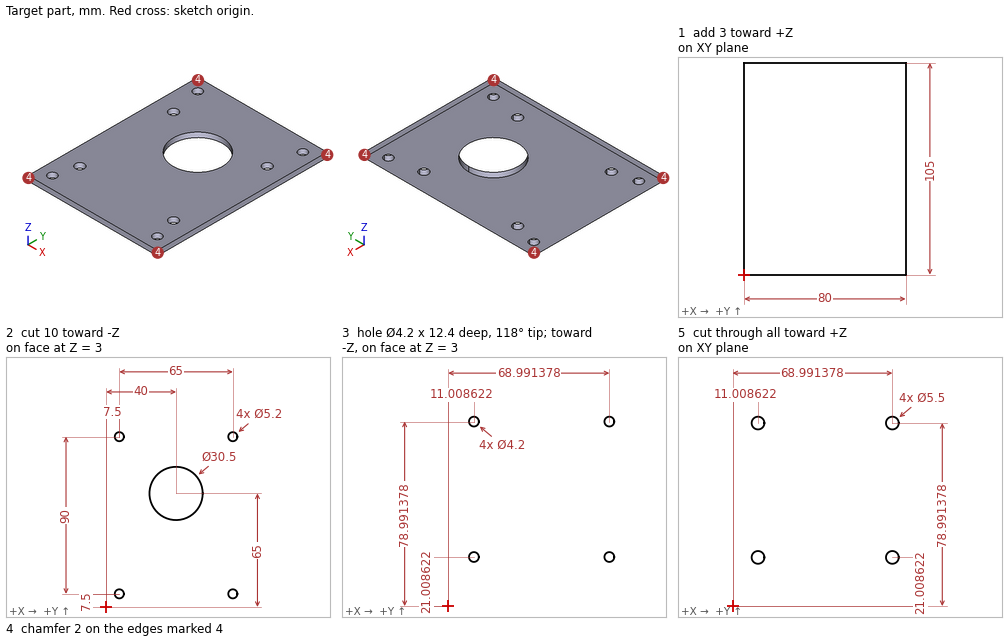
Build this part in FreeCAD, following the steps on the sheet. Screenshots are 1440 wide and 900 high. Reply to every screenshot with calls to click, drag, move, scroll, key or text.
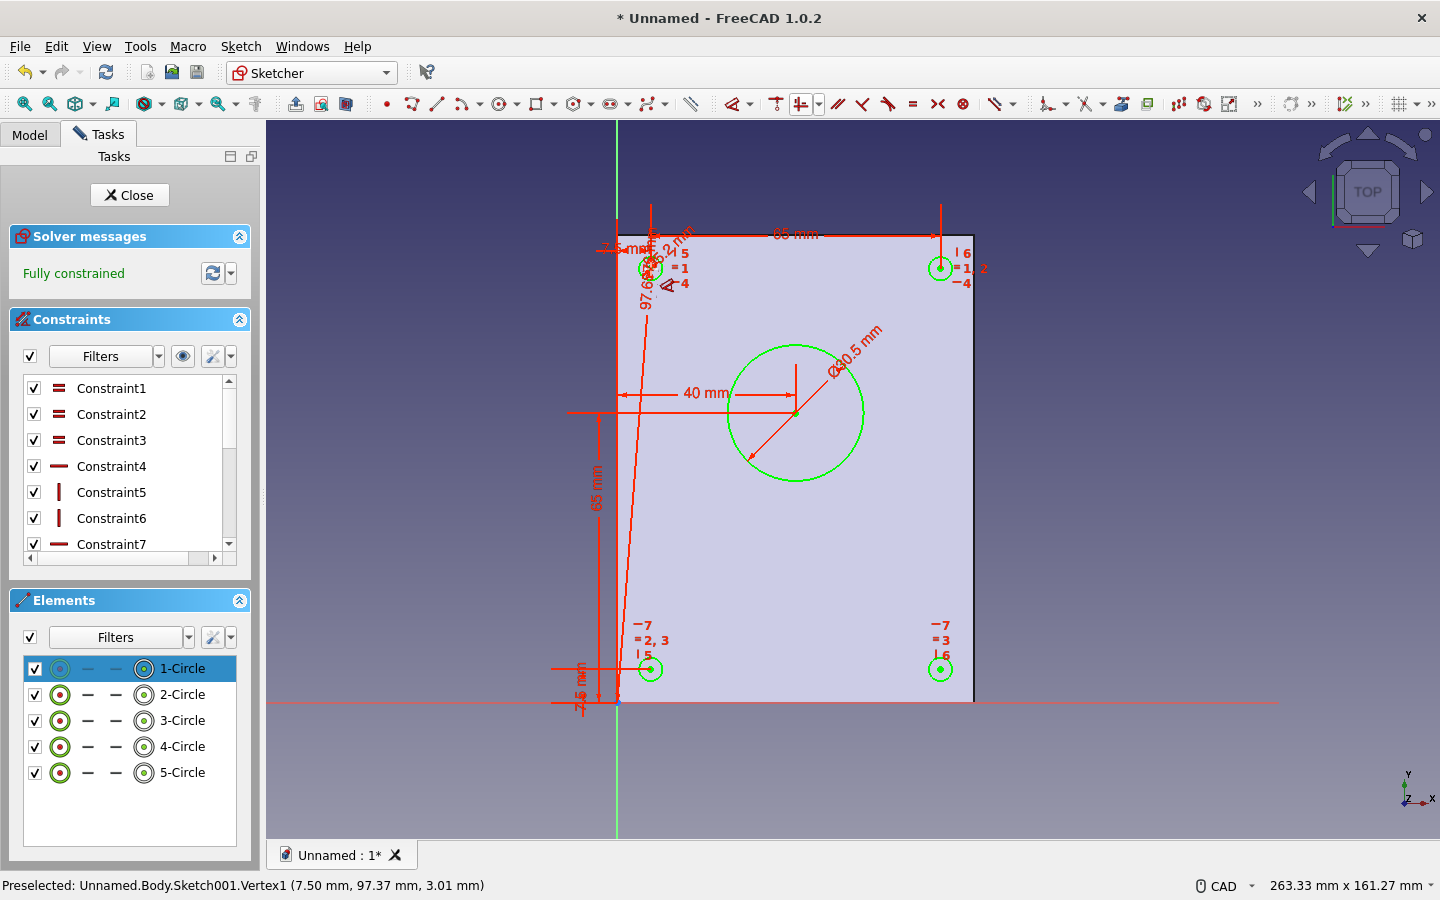
click(651, 669)
click(685, 469)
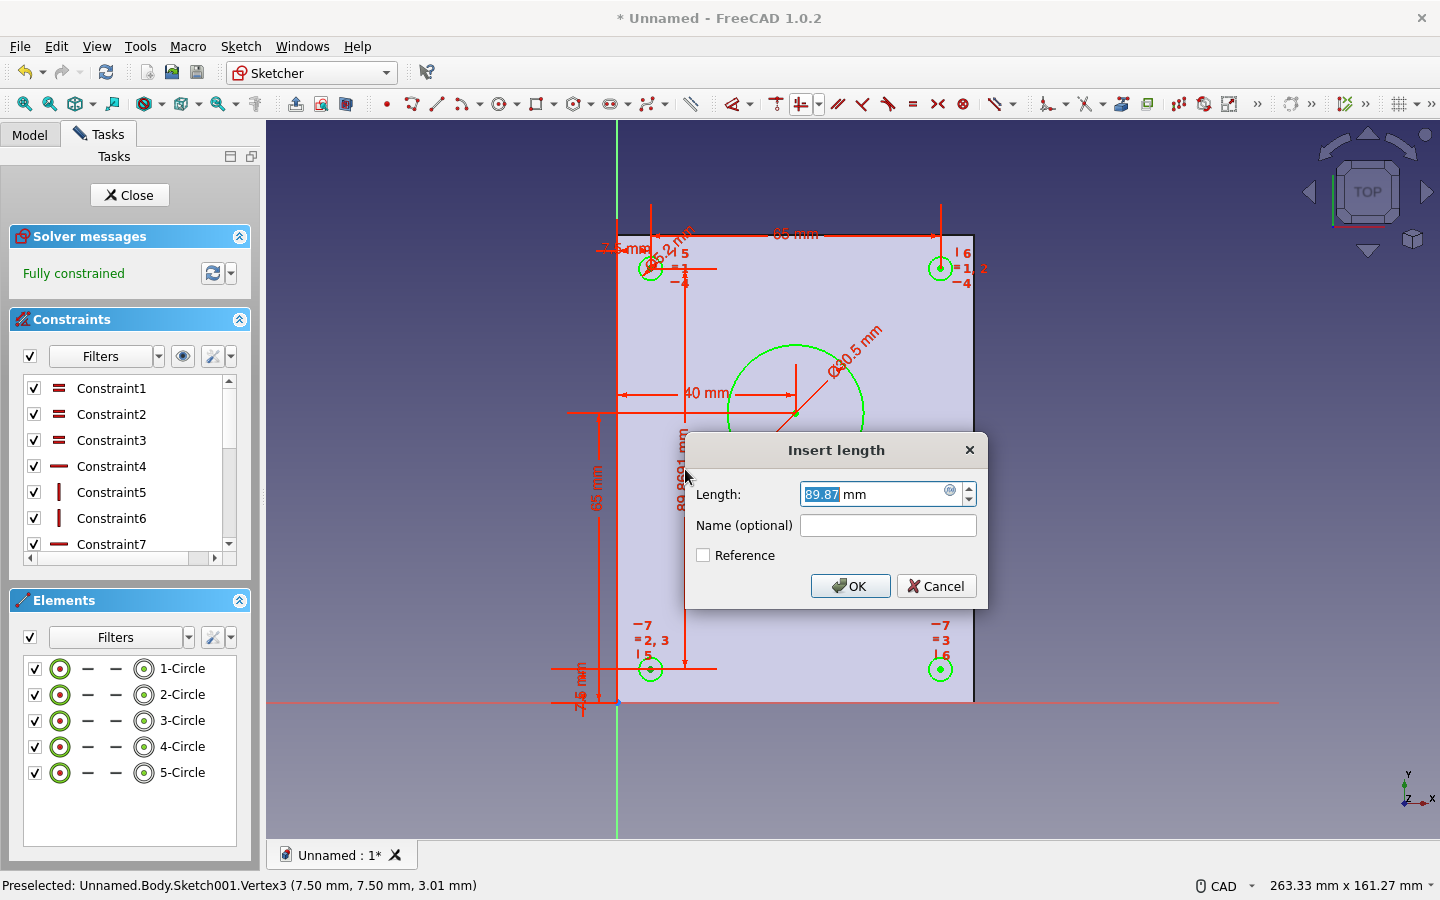
text(90)
key(Return)
key(Escape)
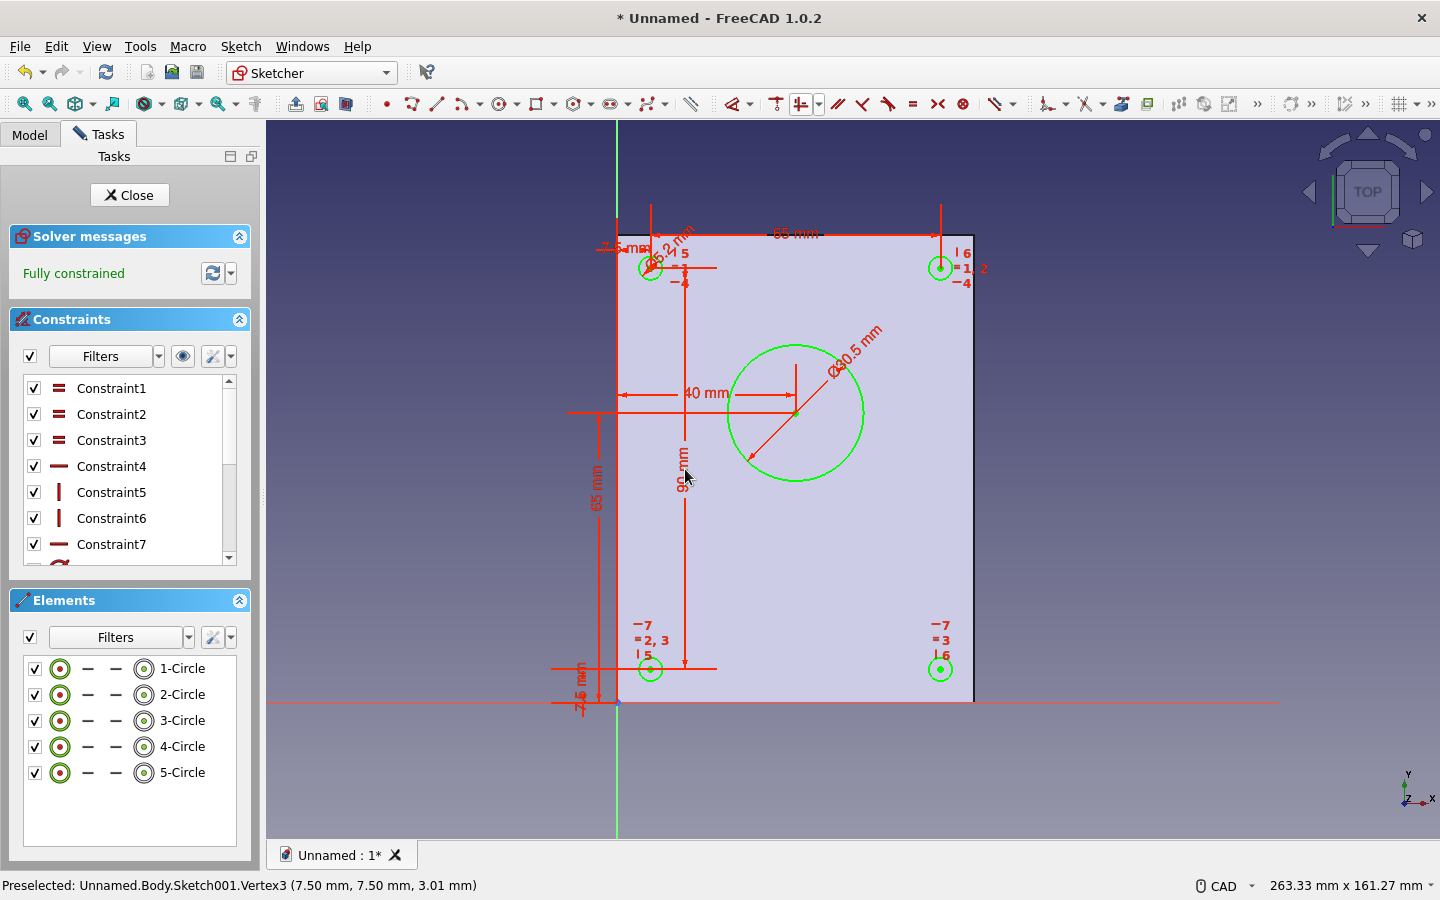
click(130, 195)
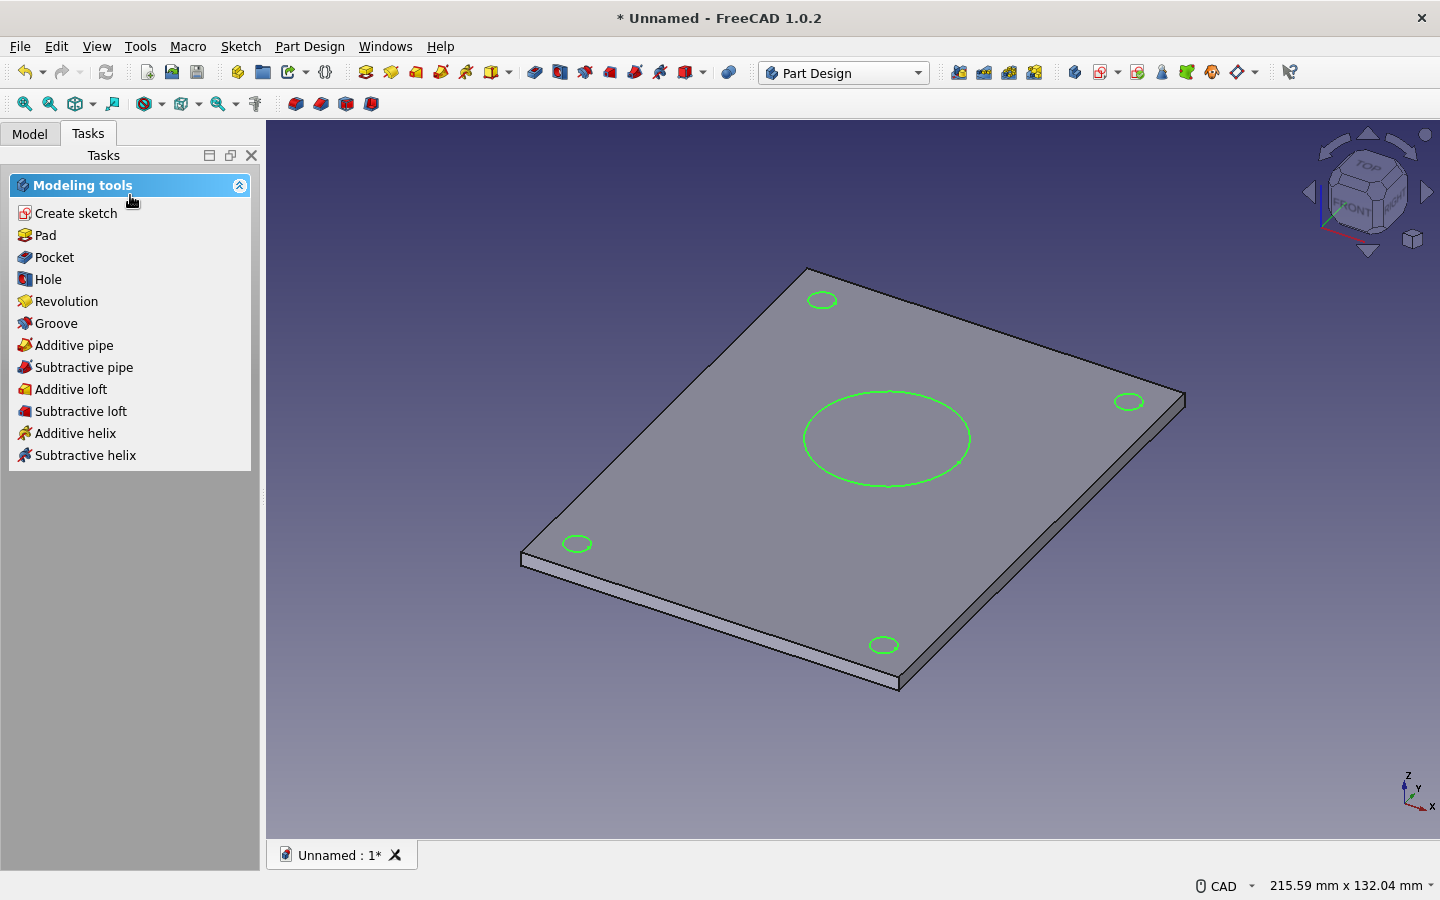
click(535, 72)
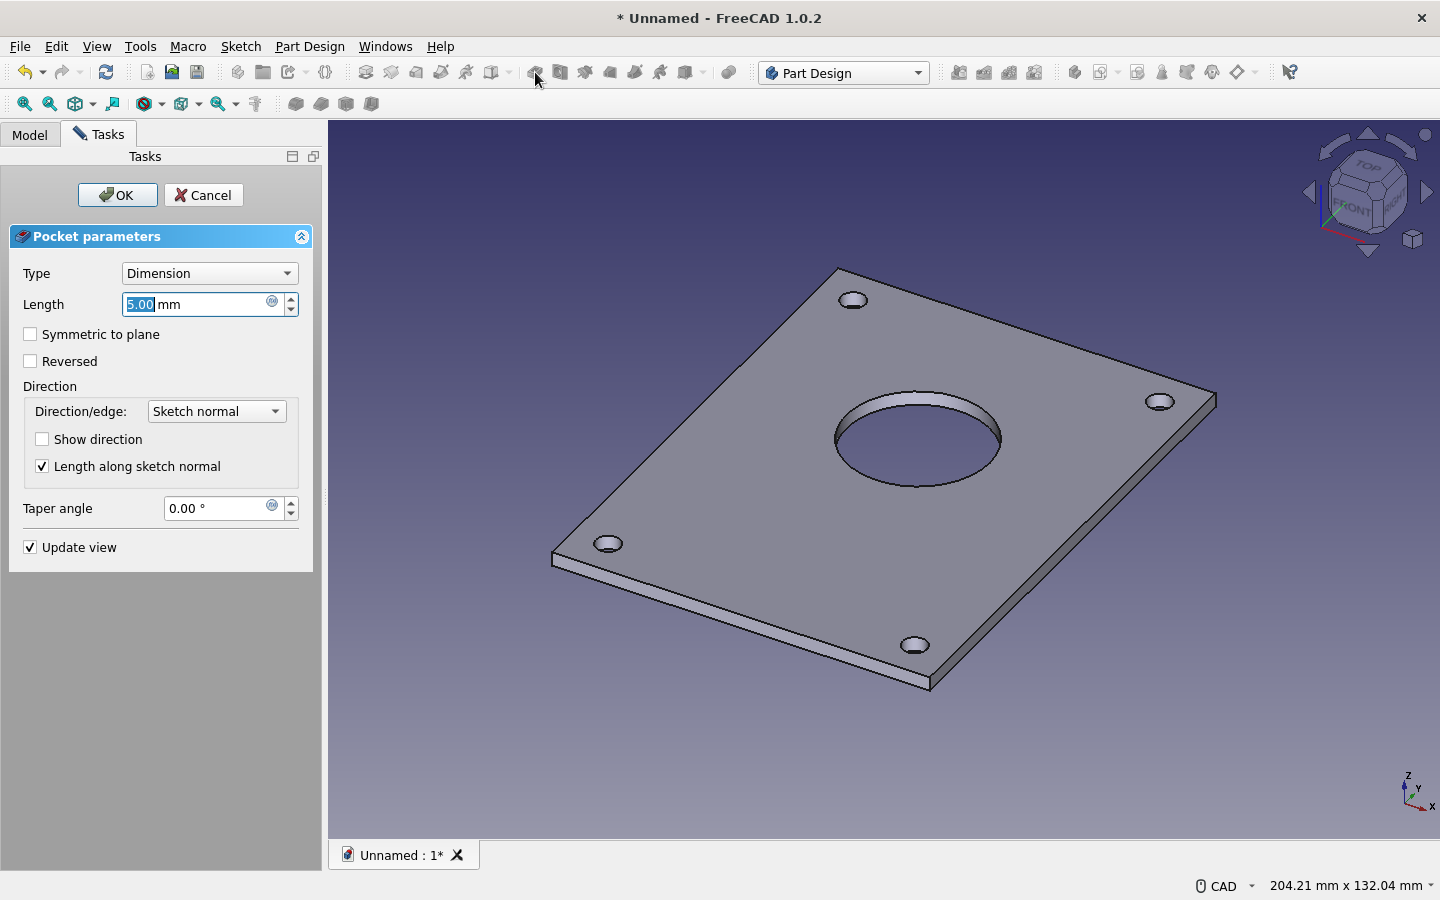
text(10)
key(Tab)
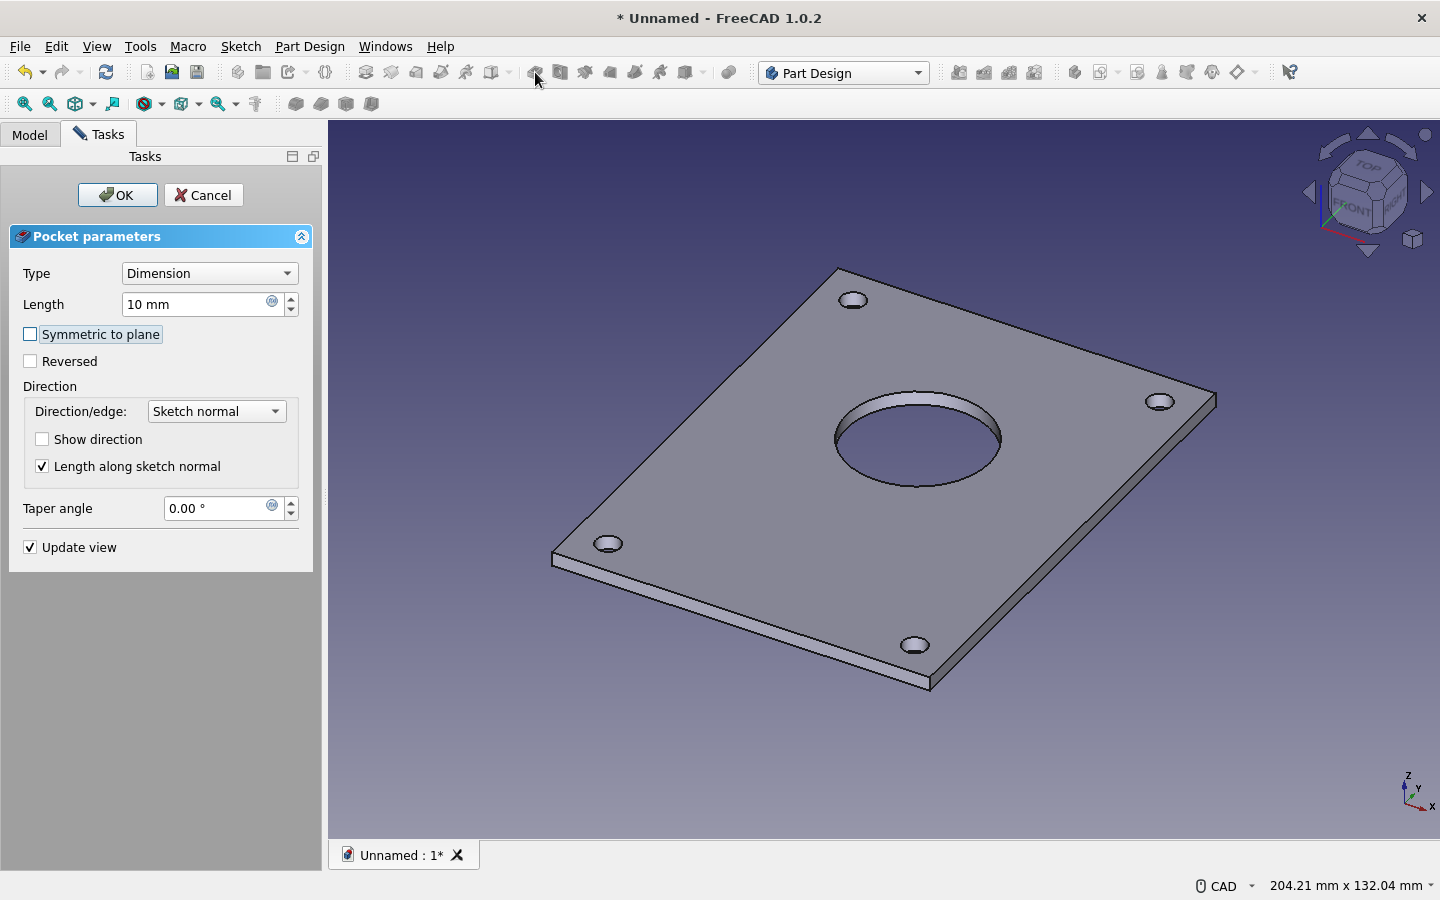
click(118, 195)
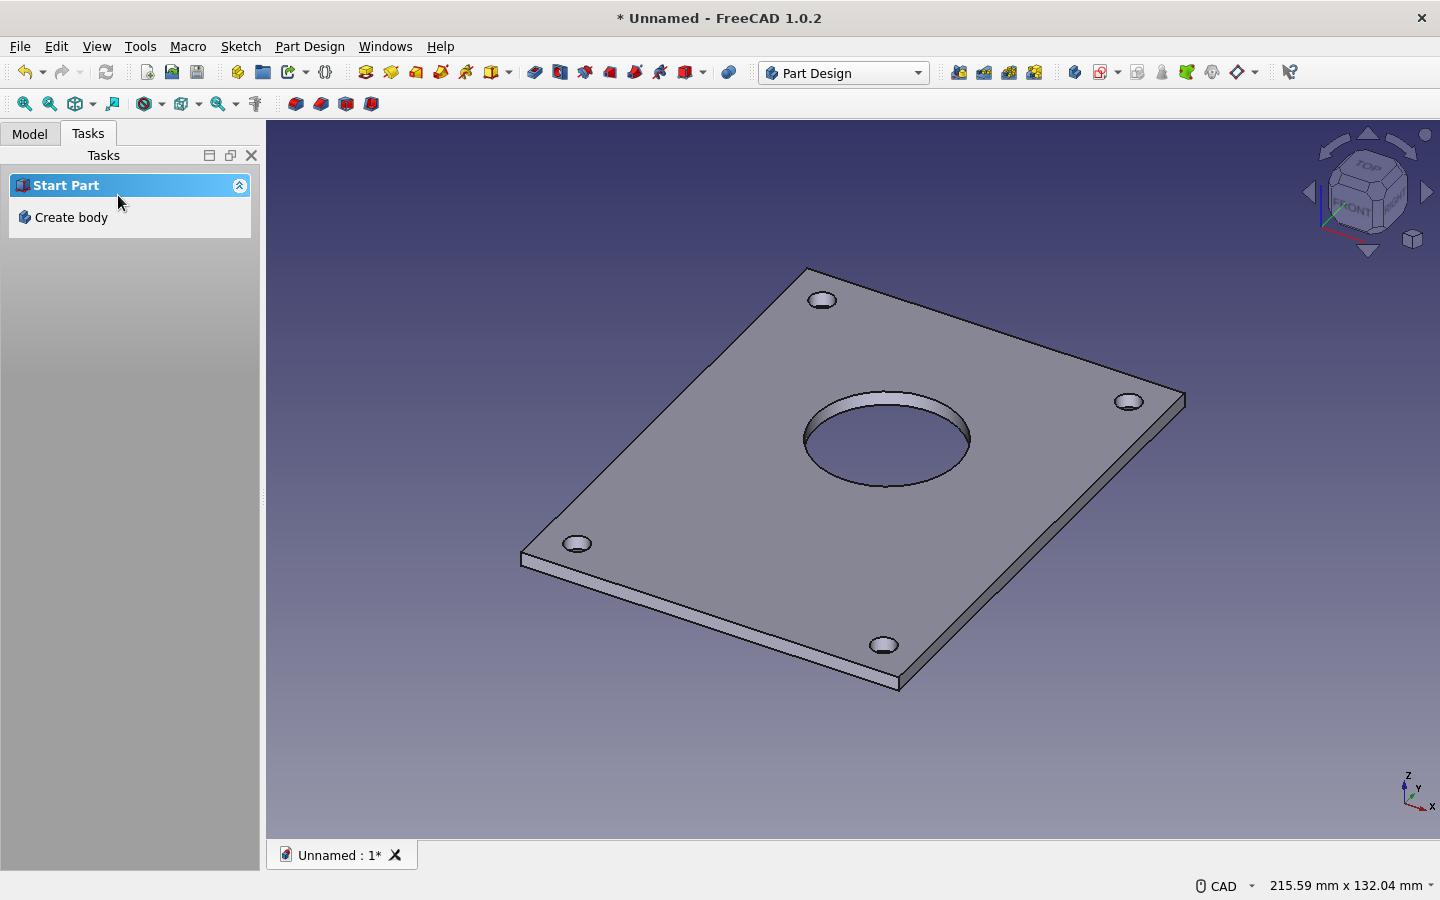
click(825, 571)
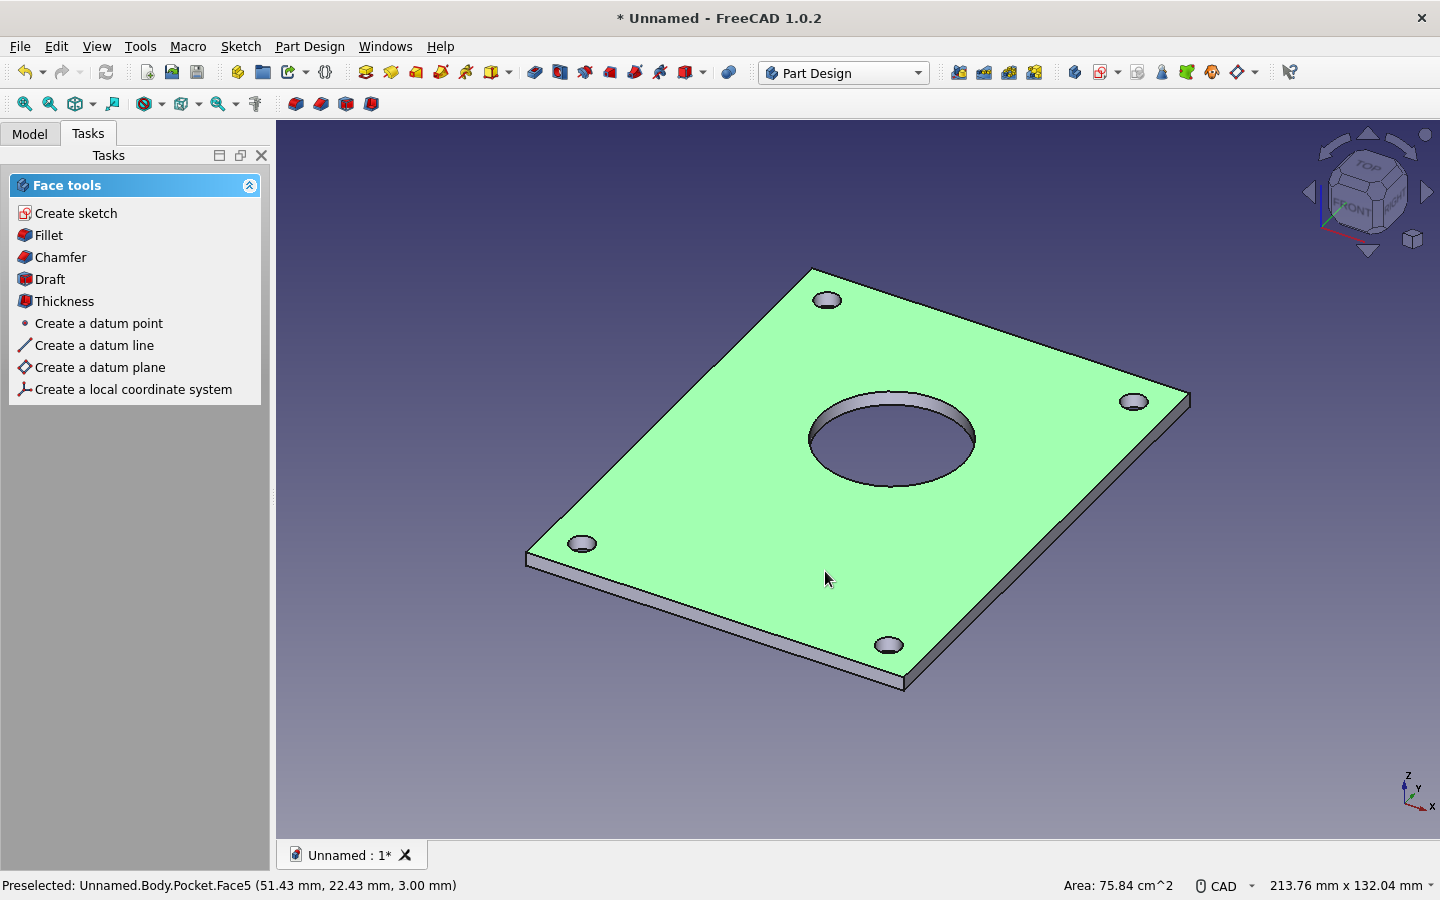
click(1100, 72)